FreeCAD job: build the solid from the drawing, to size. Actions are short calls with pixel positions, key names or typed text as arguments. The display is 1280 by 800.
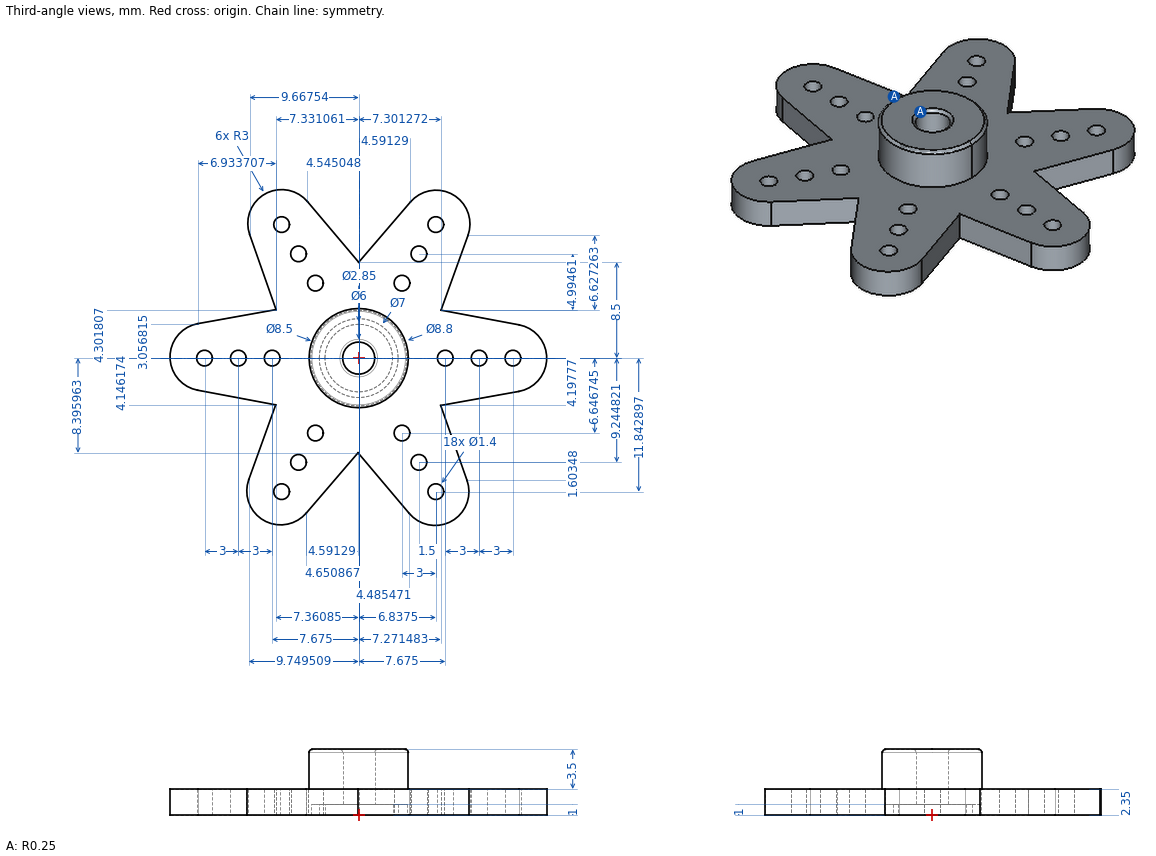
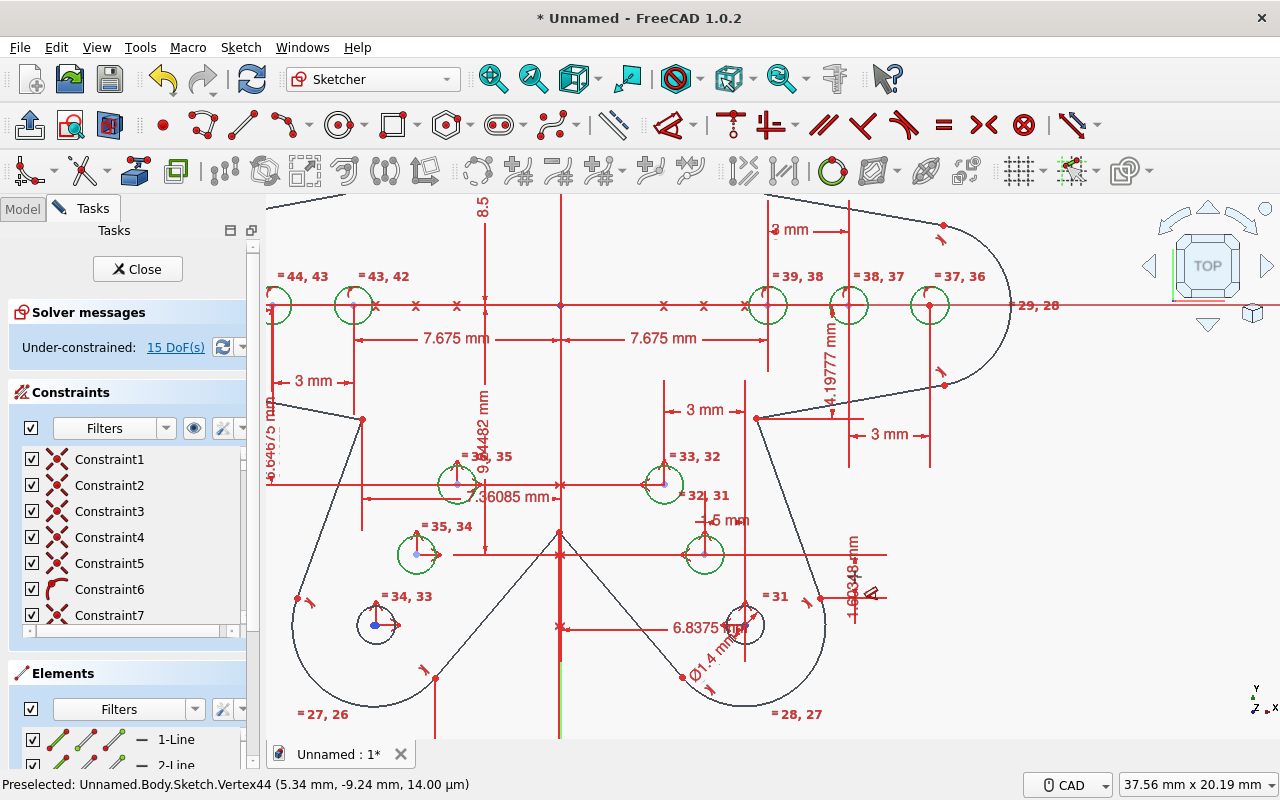
scroll(822, 599, down, 4)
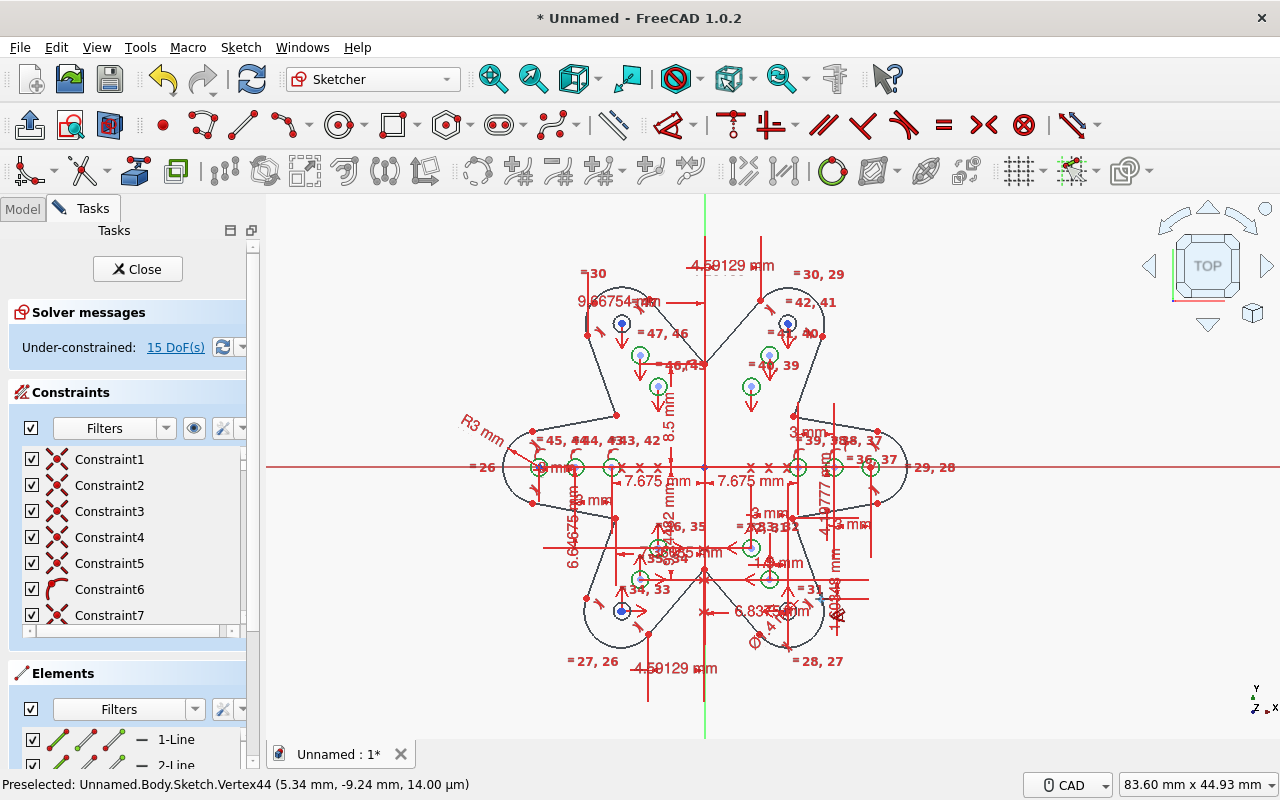
click(794, 417)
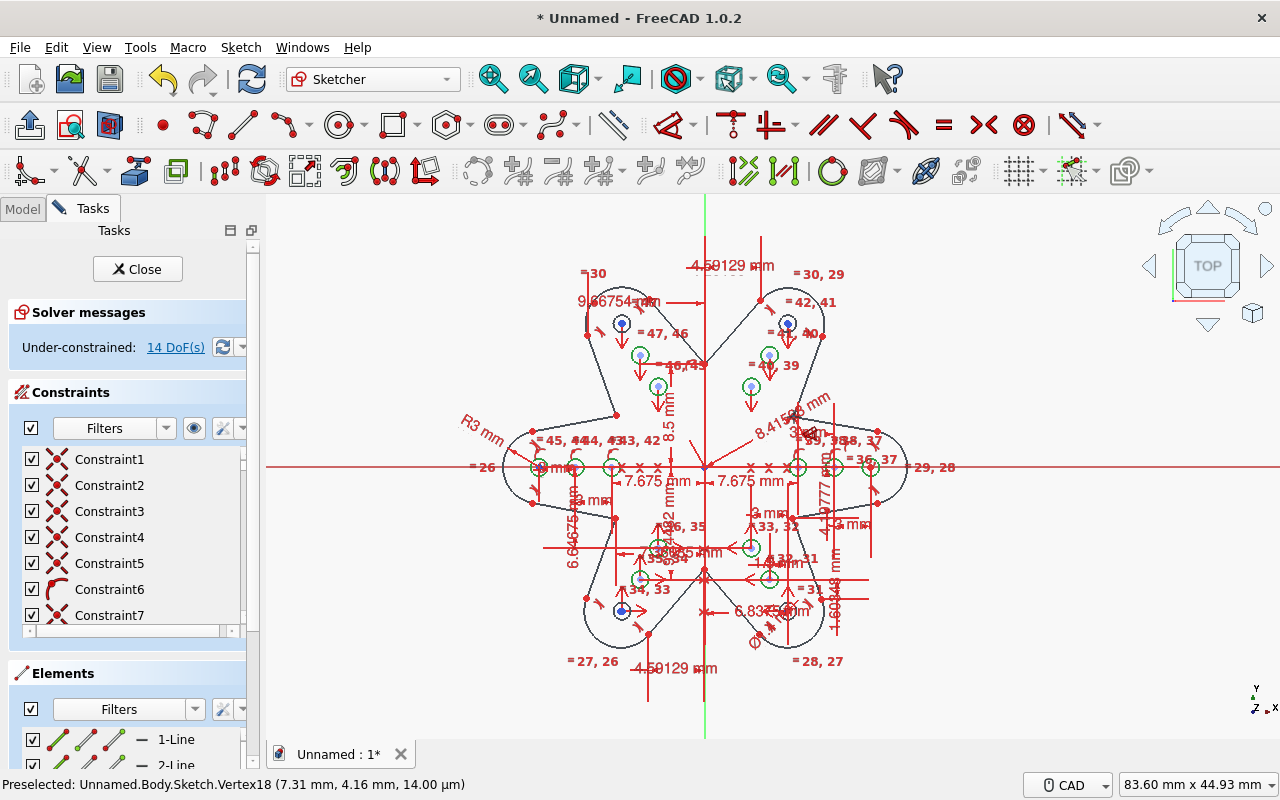
click(770, 355)
click(828, 386)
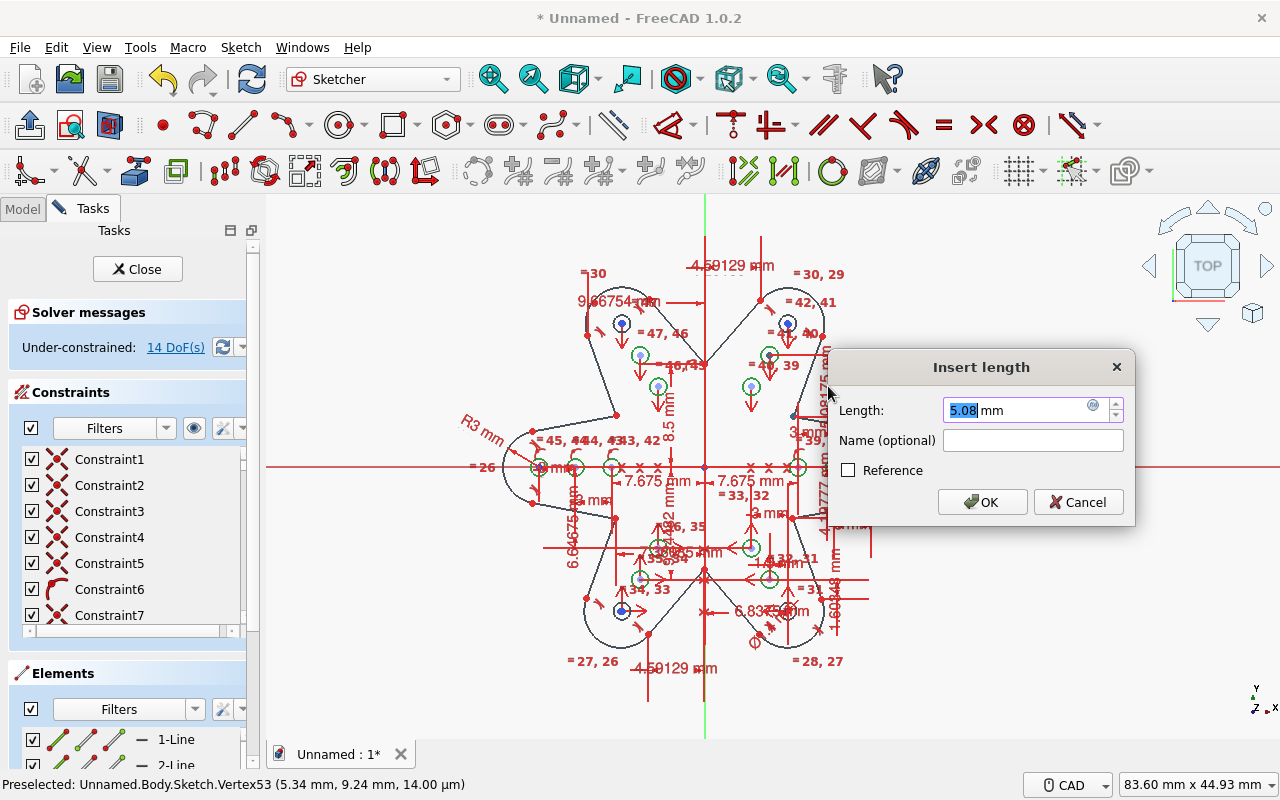
text(4.99461)
key(Return)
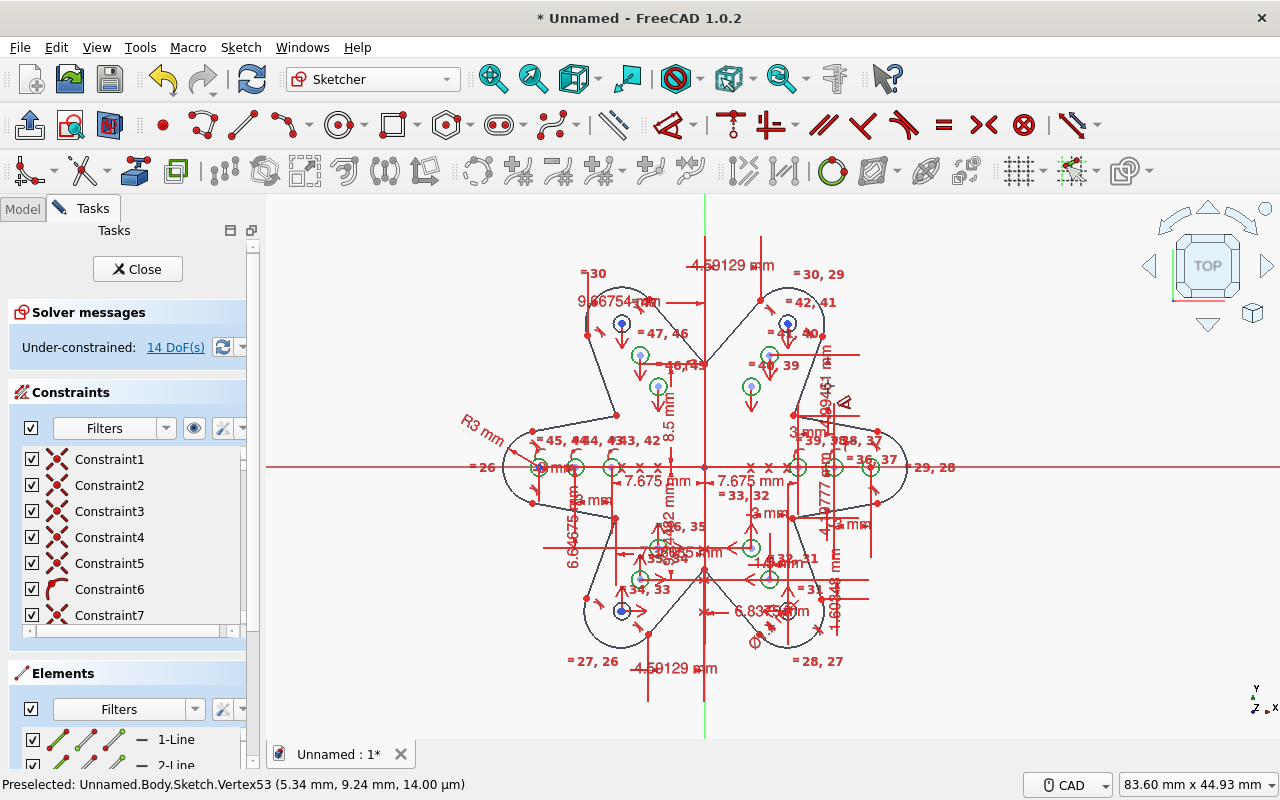
click(616, 416)
click(681, 382)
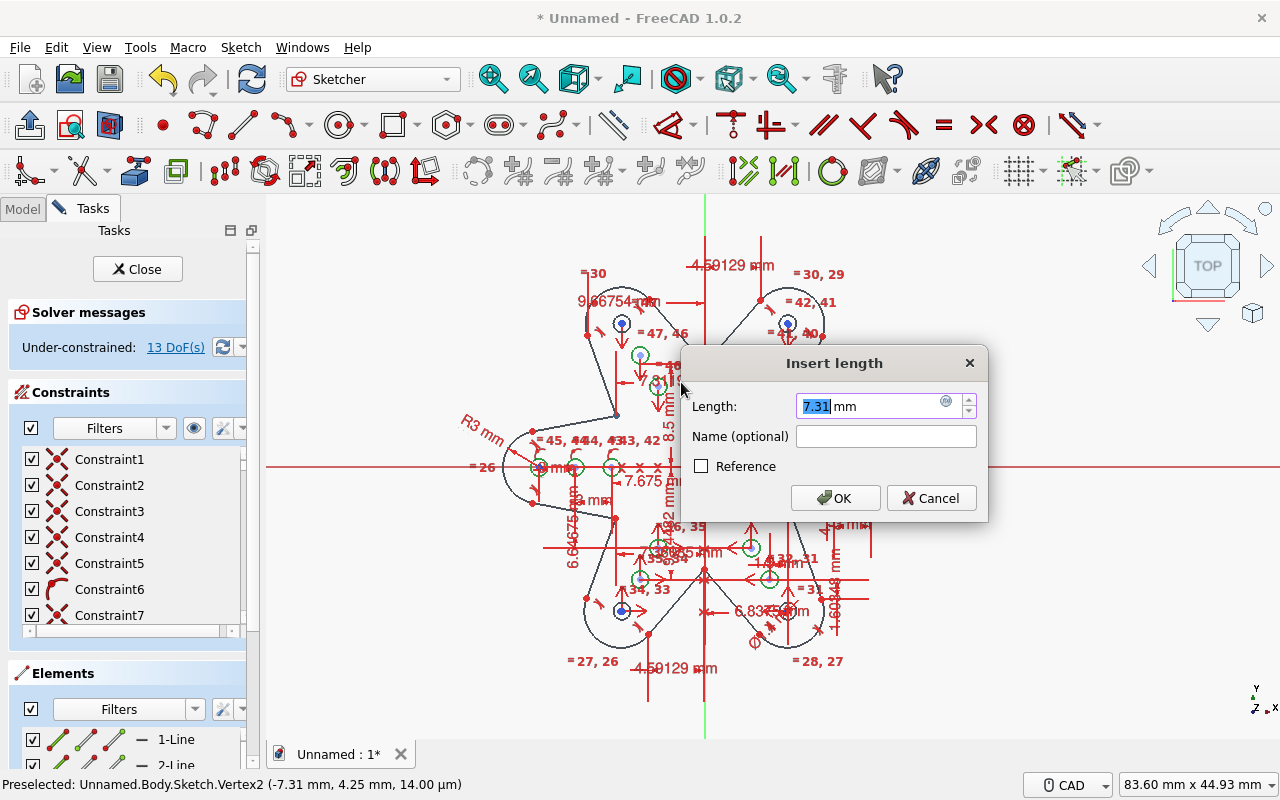
text(7.331061)
key(Return)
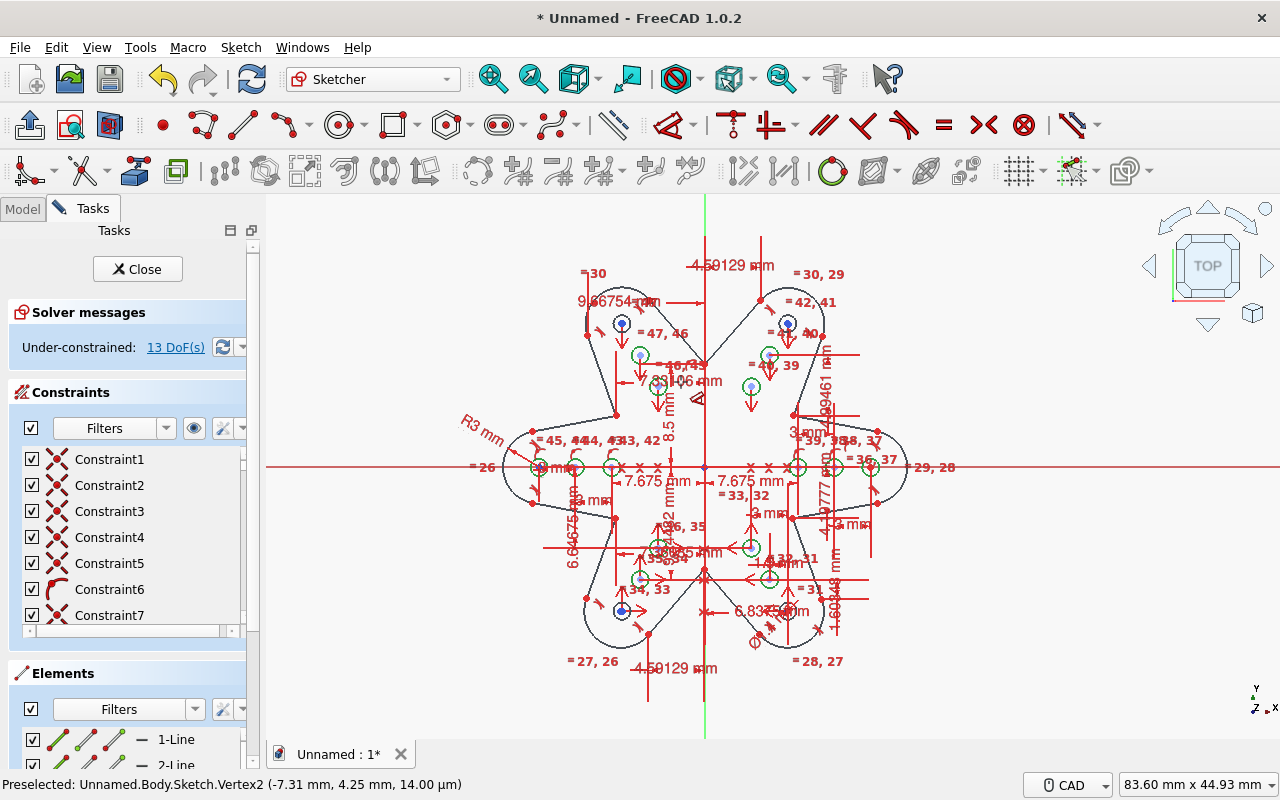
click(616, 416)
click(582, 442)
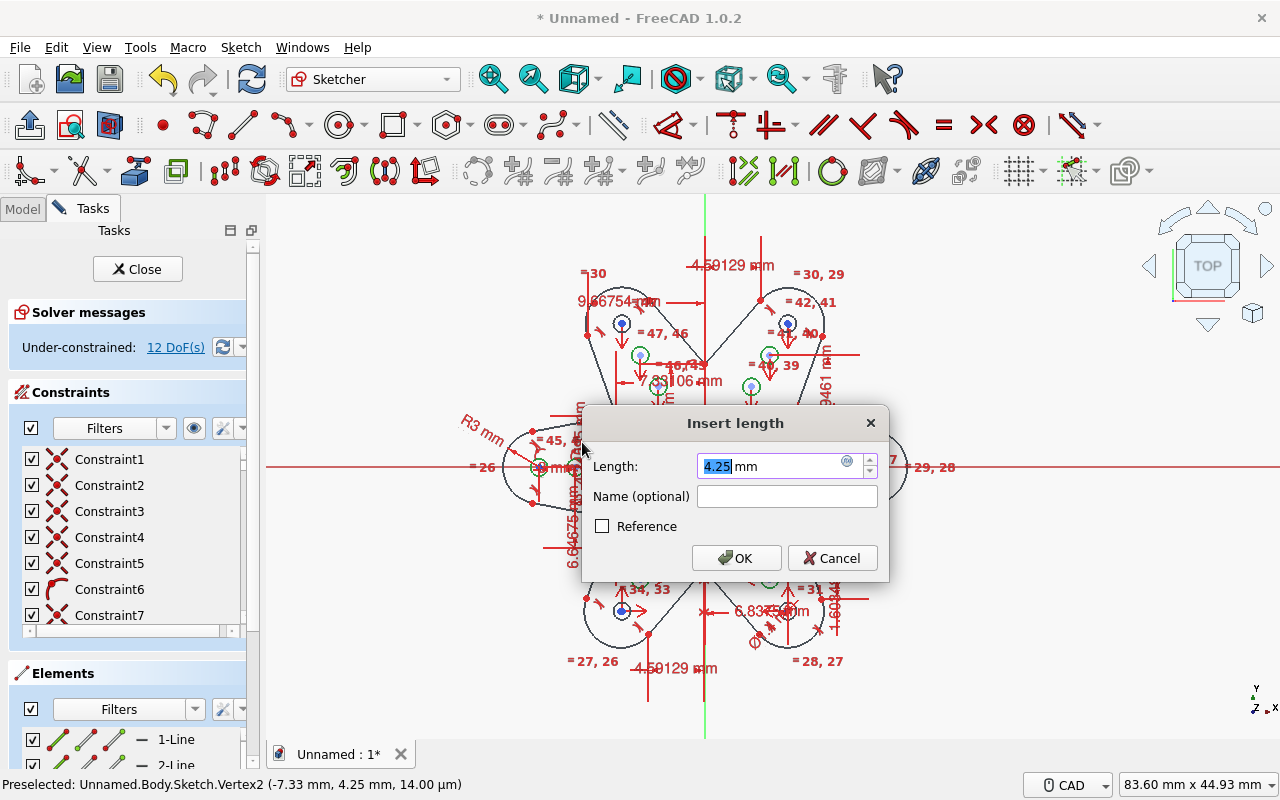
text(4.301807)
key(Return)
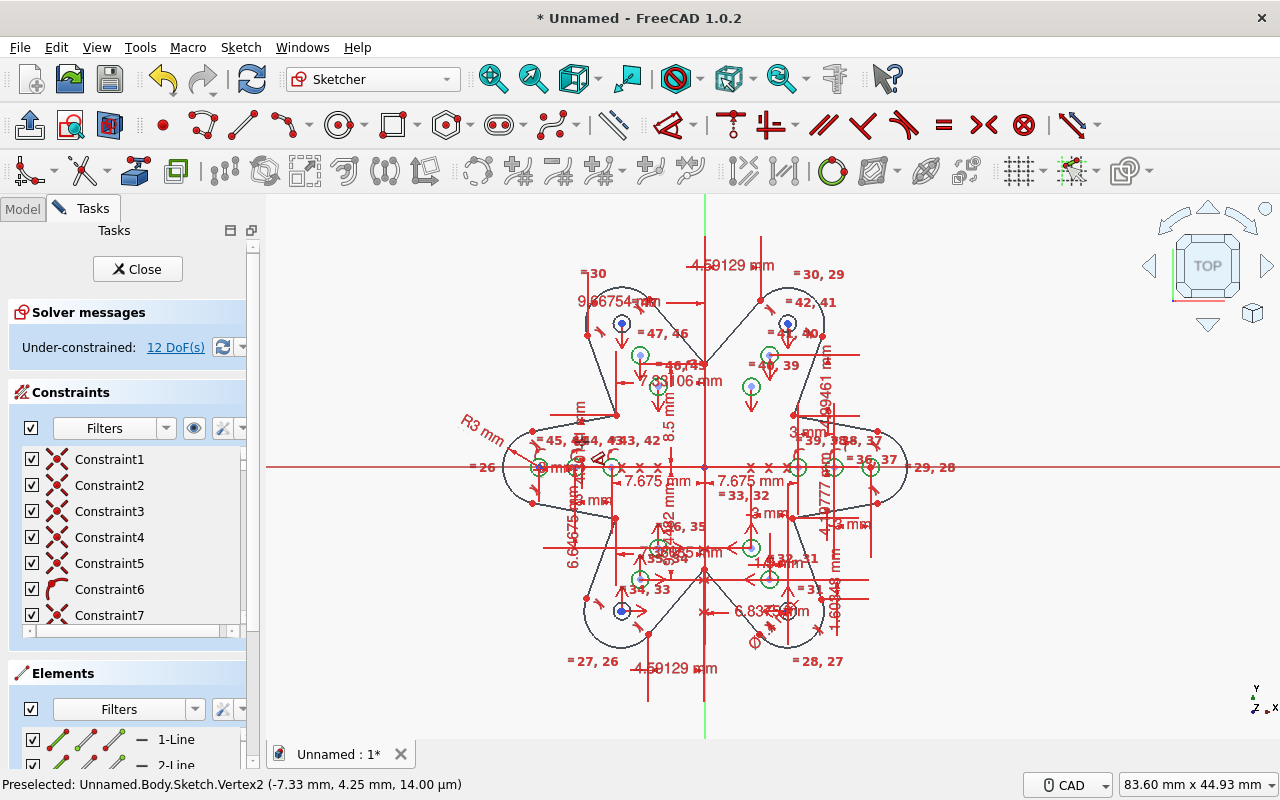
click(532, 432)
click(402, 450)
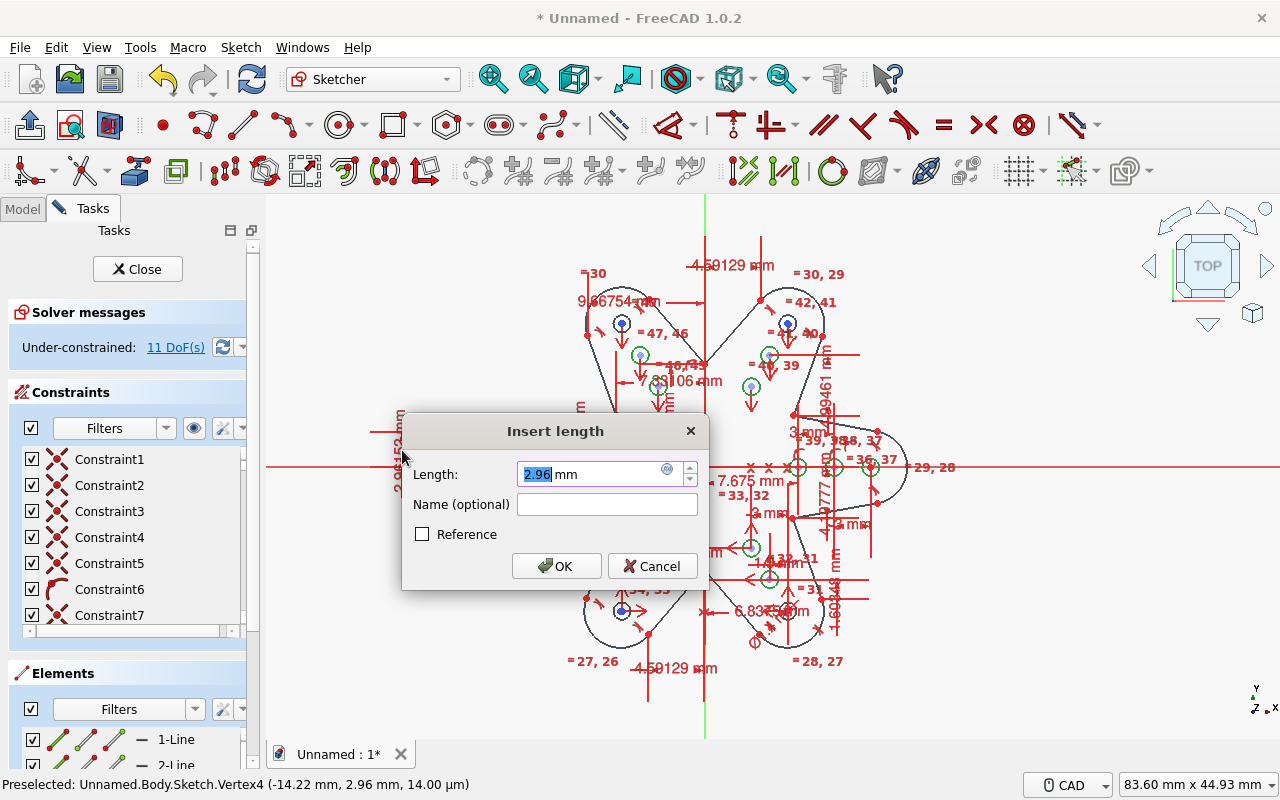
text(3.056815)
key(Return)